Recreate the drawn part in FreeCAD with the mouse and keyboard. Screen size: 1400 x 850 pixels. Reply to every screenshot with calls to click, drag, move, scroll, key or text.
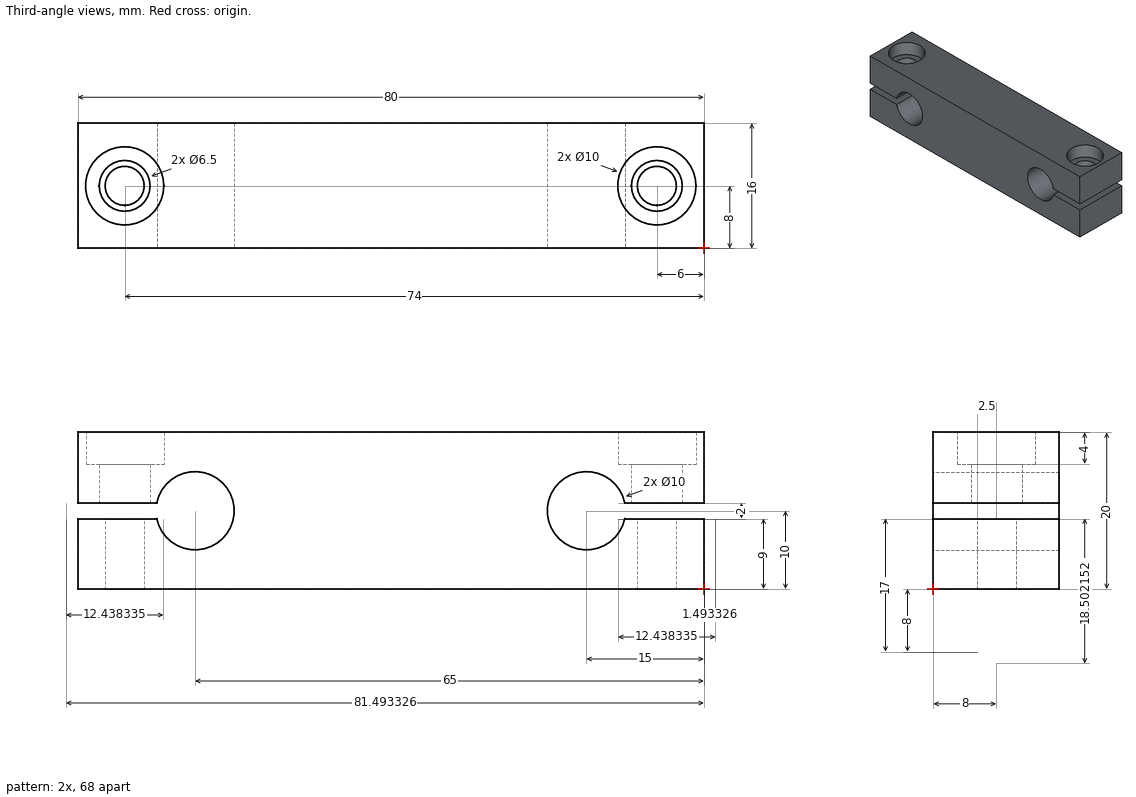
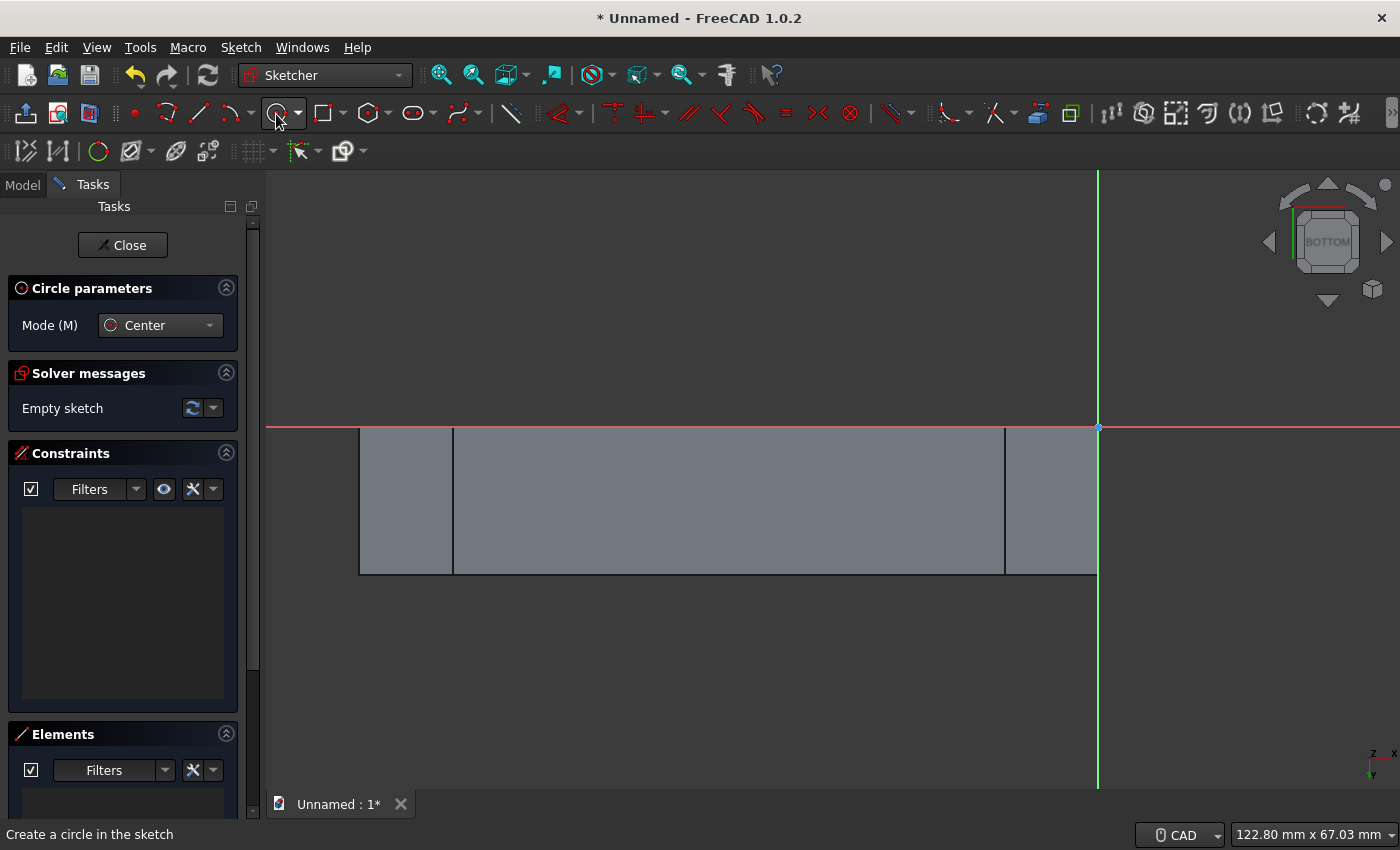
click(415, 501)
click(436, 480)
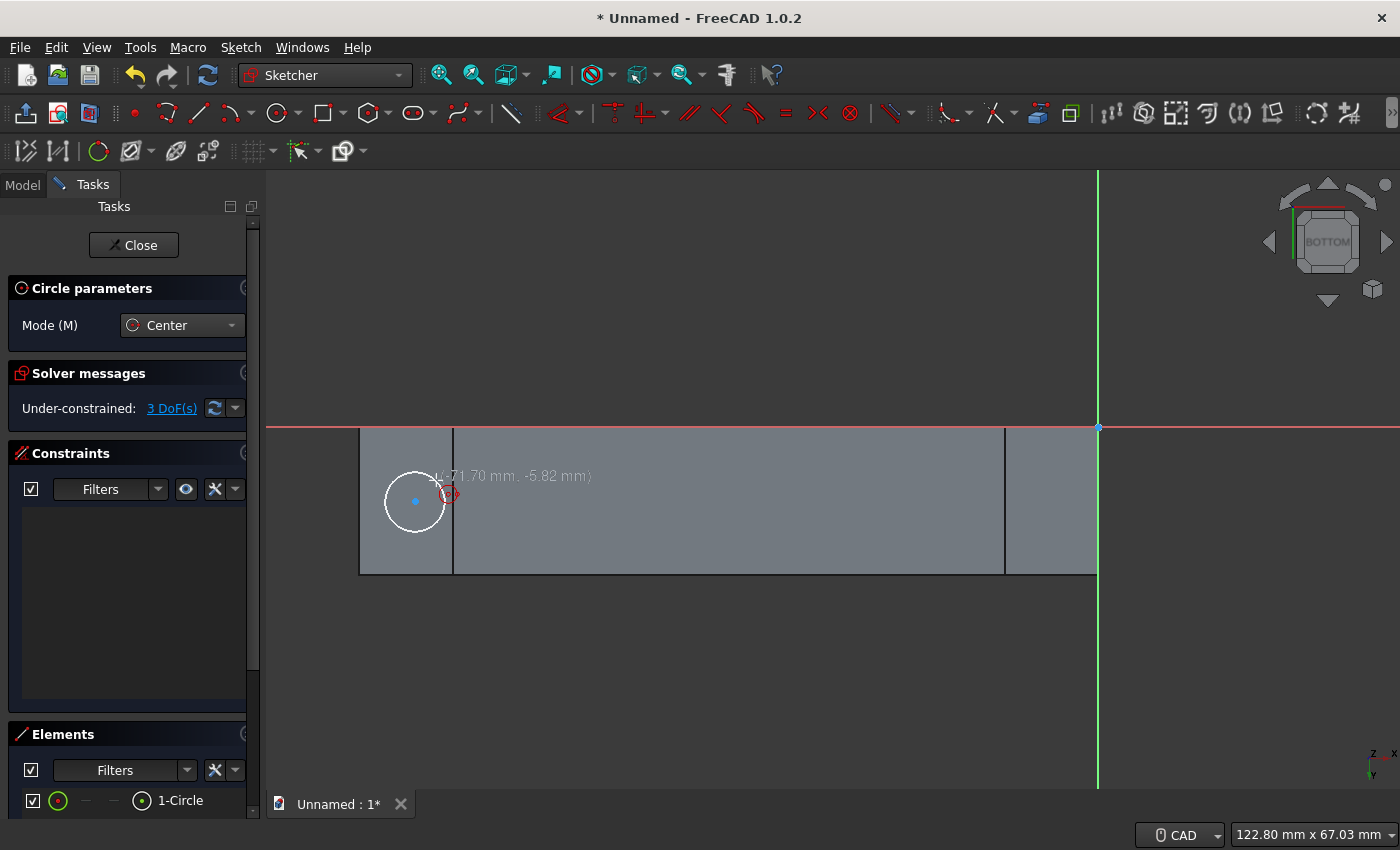
click(1043, 501)
click(1064, 480)
key(Escape)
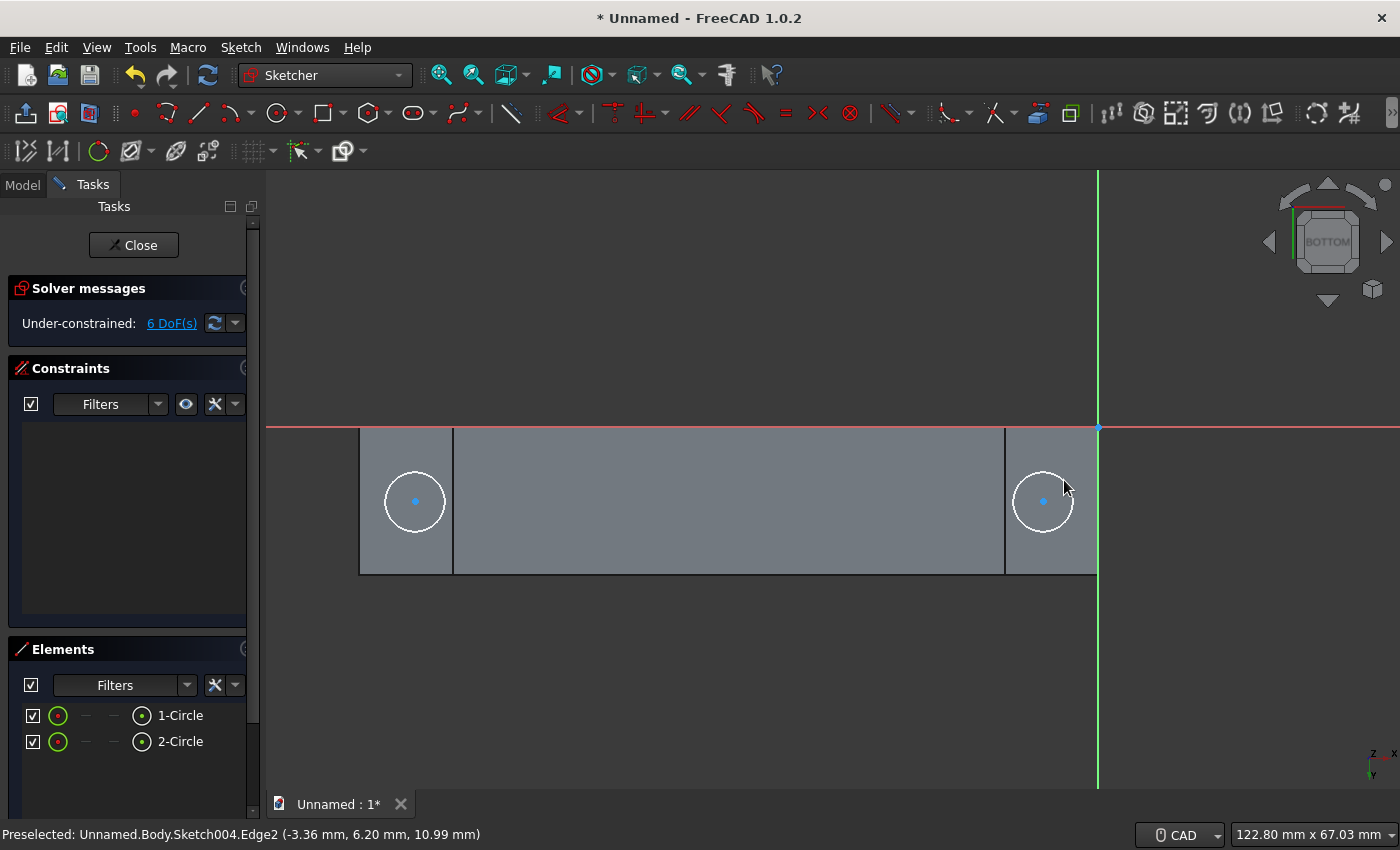
click(436, 481)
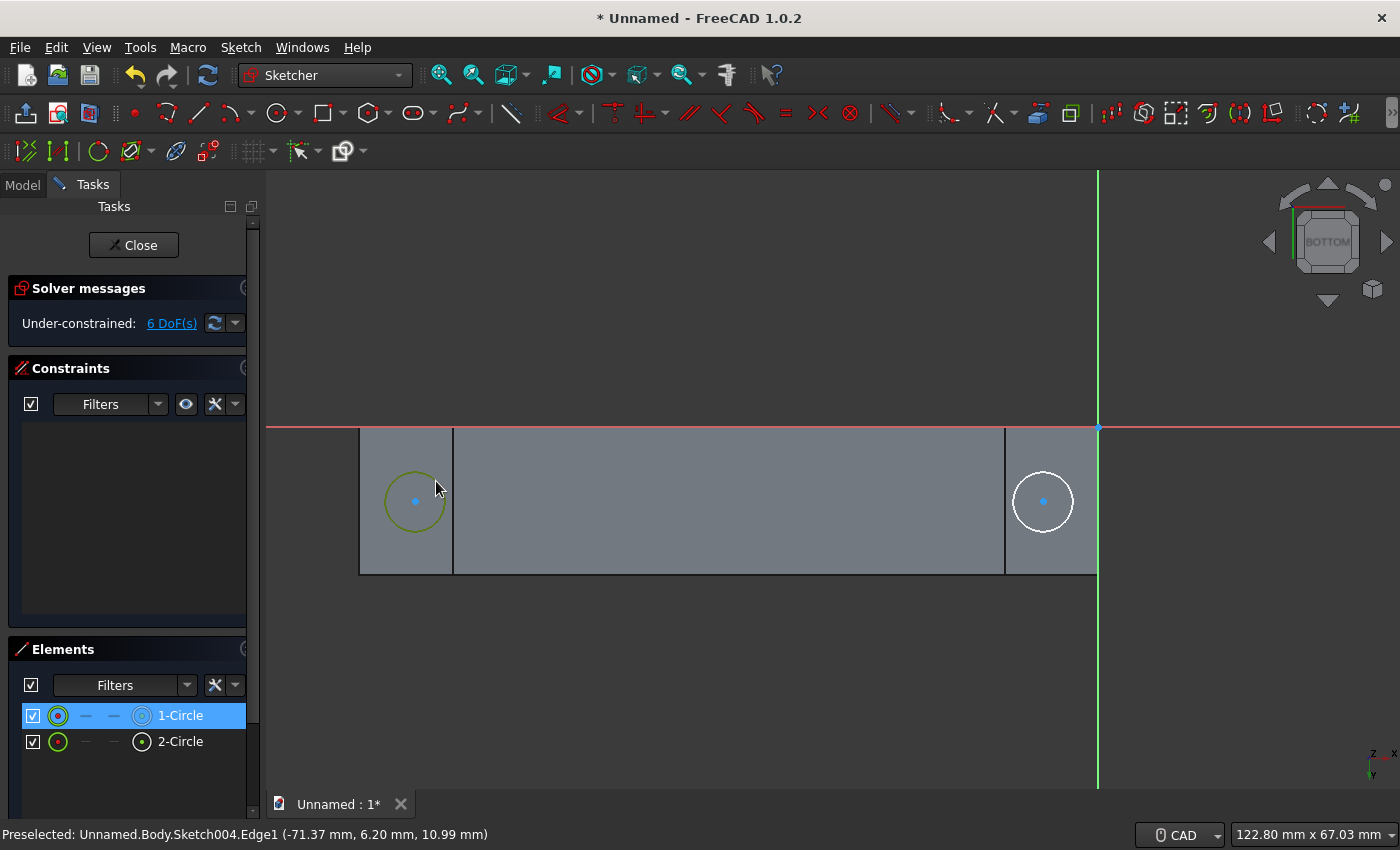
click(1064, 481)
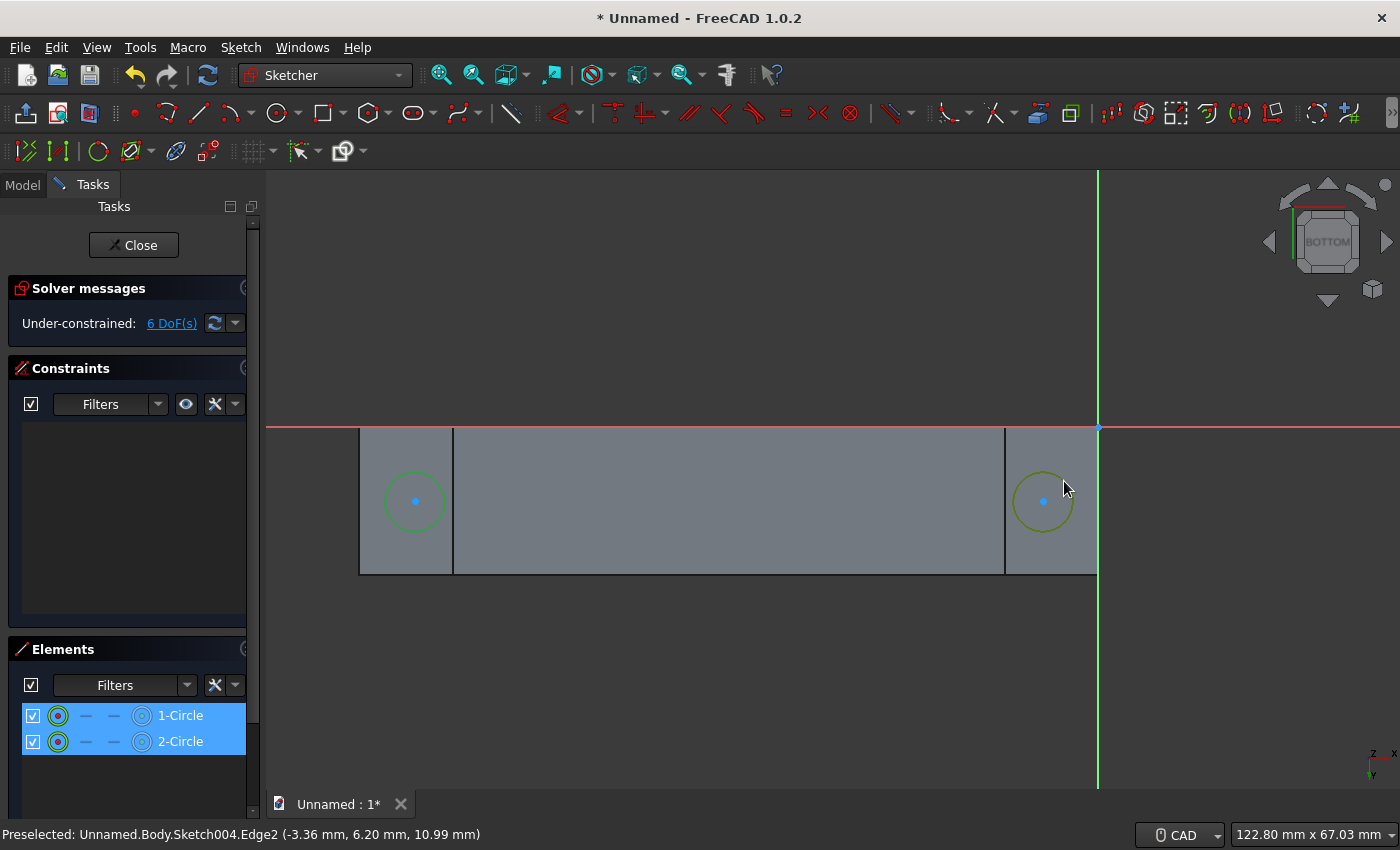
click(786, 114)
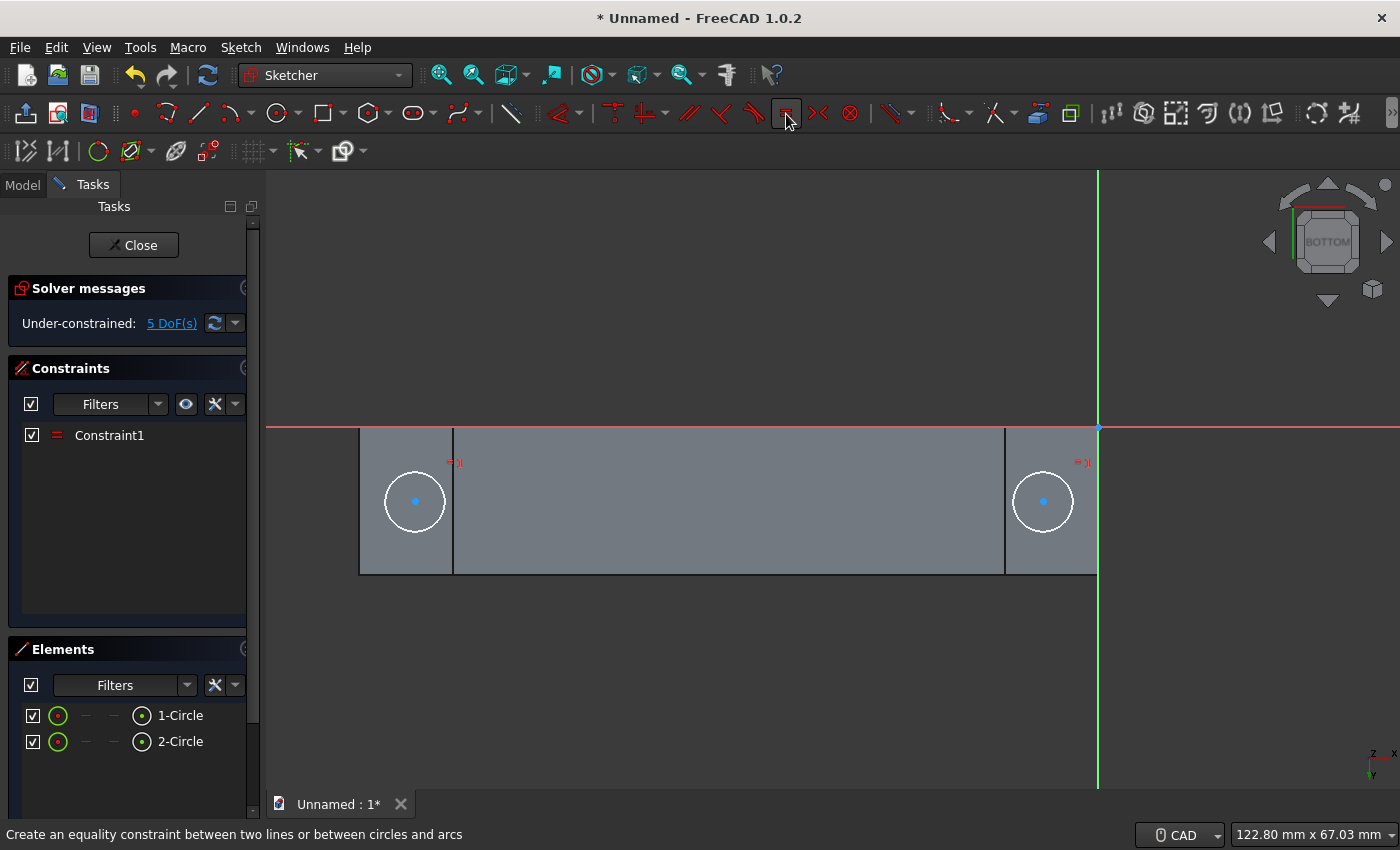
click(558, 114)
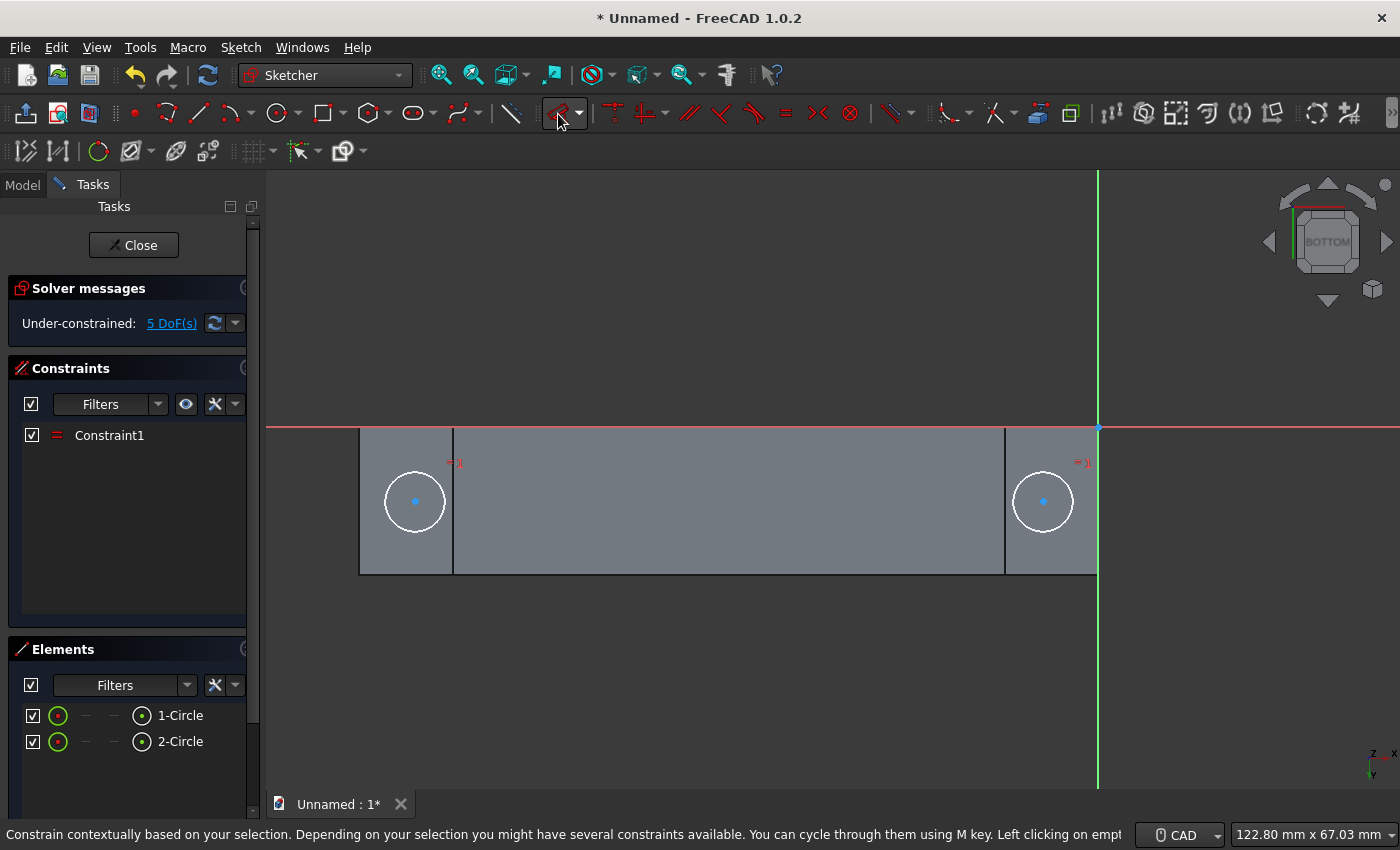
click(436, 481)
click(459, 458)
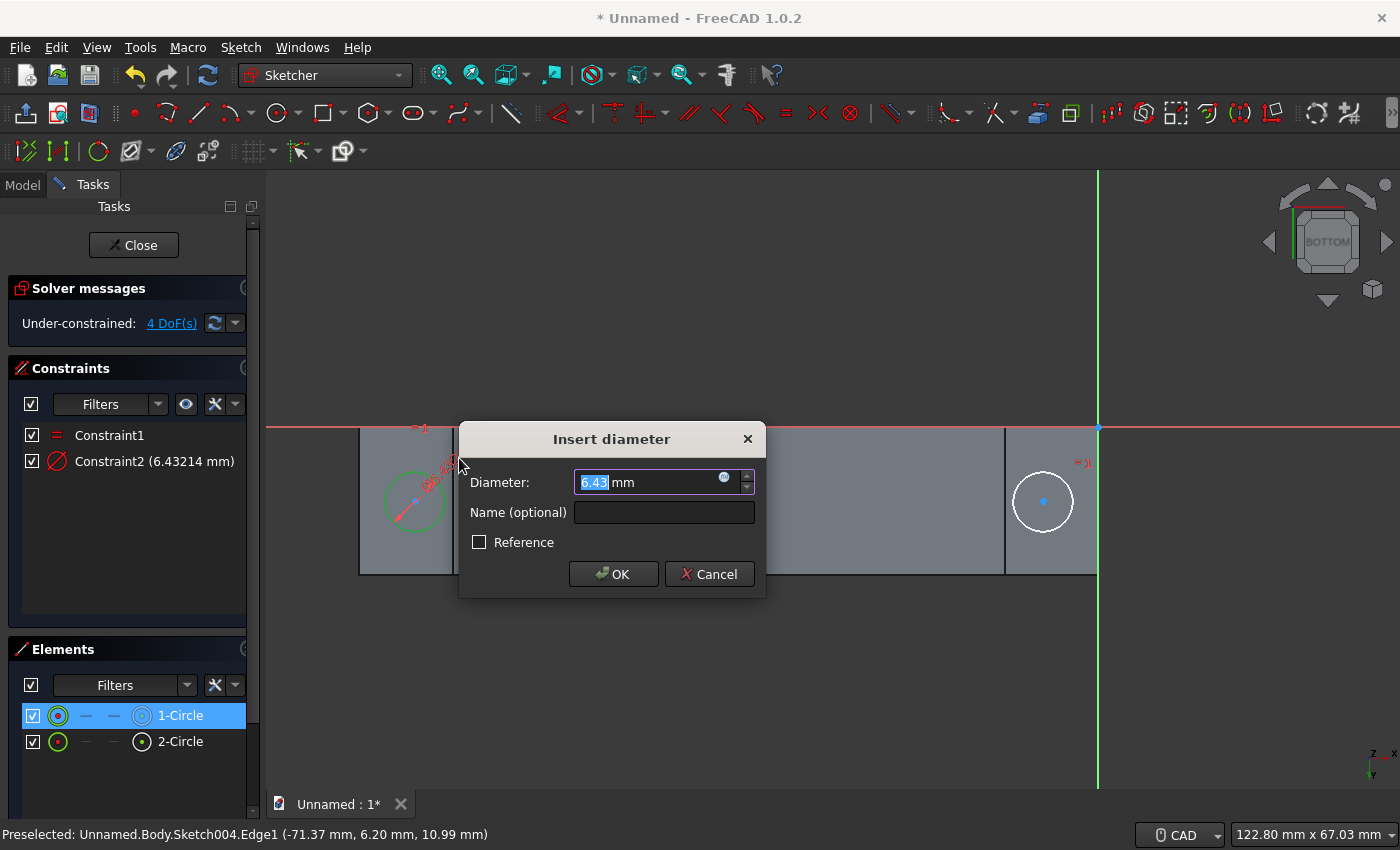
text(6.5)
key(Return)